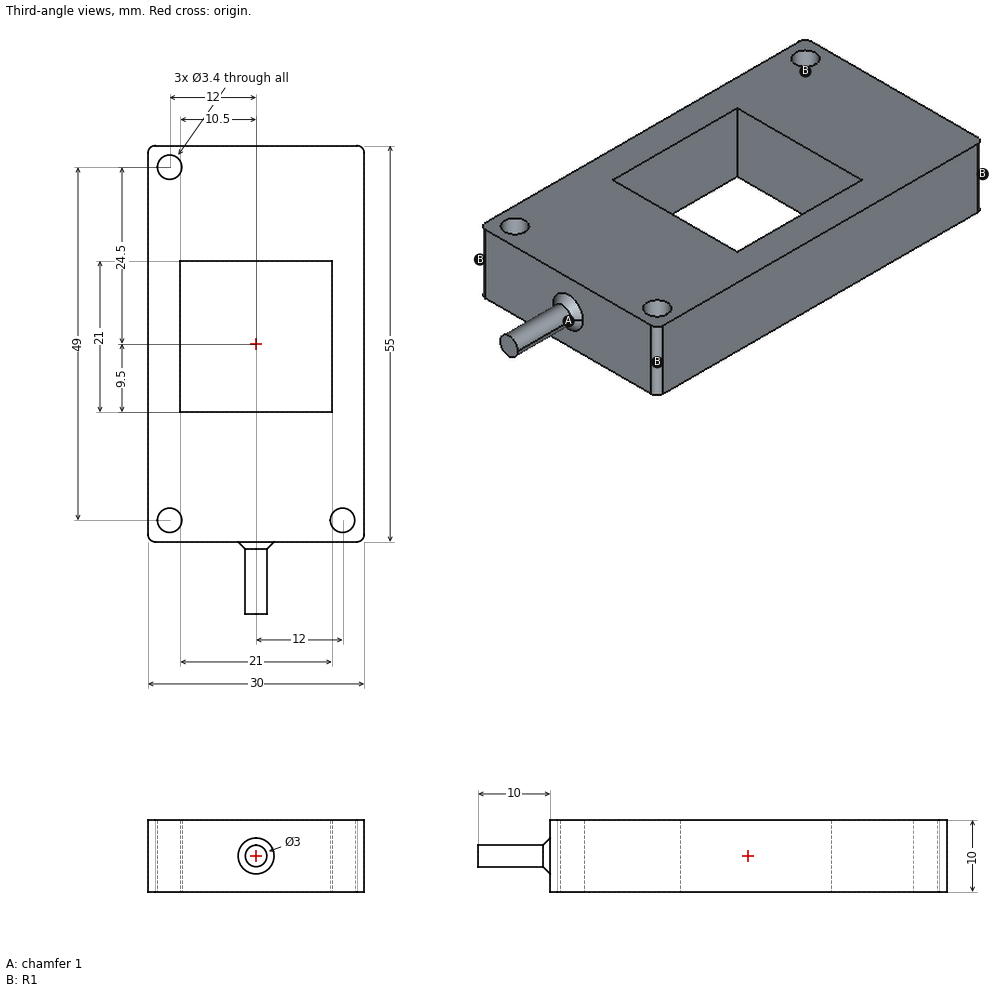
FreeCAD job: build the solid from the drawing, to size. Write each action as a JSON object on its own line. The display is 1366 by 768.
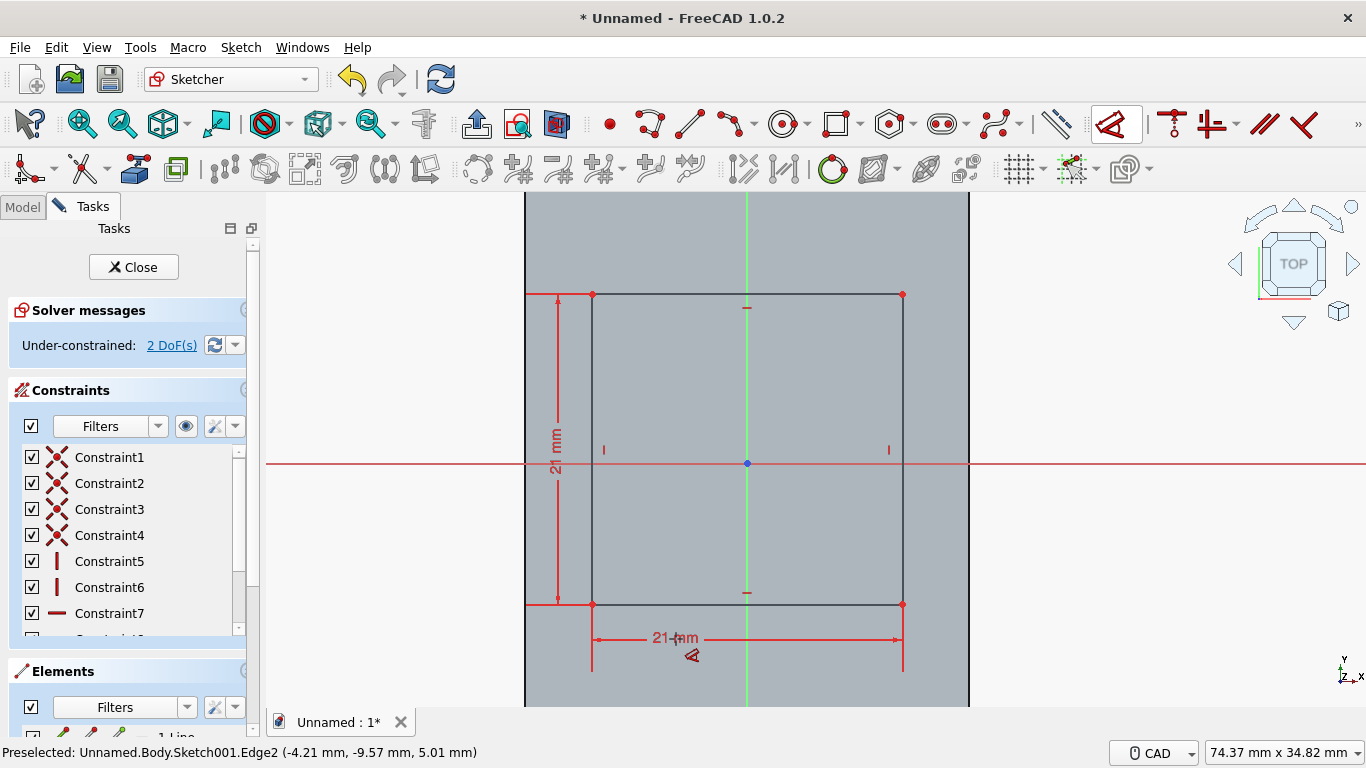
{"action": "left_click", "coordinate": [592, 605]}
{"action": "left_click", "coordinate": [558, 534]}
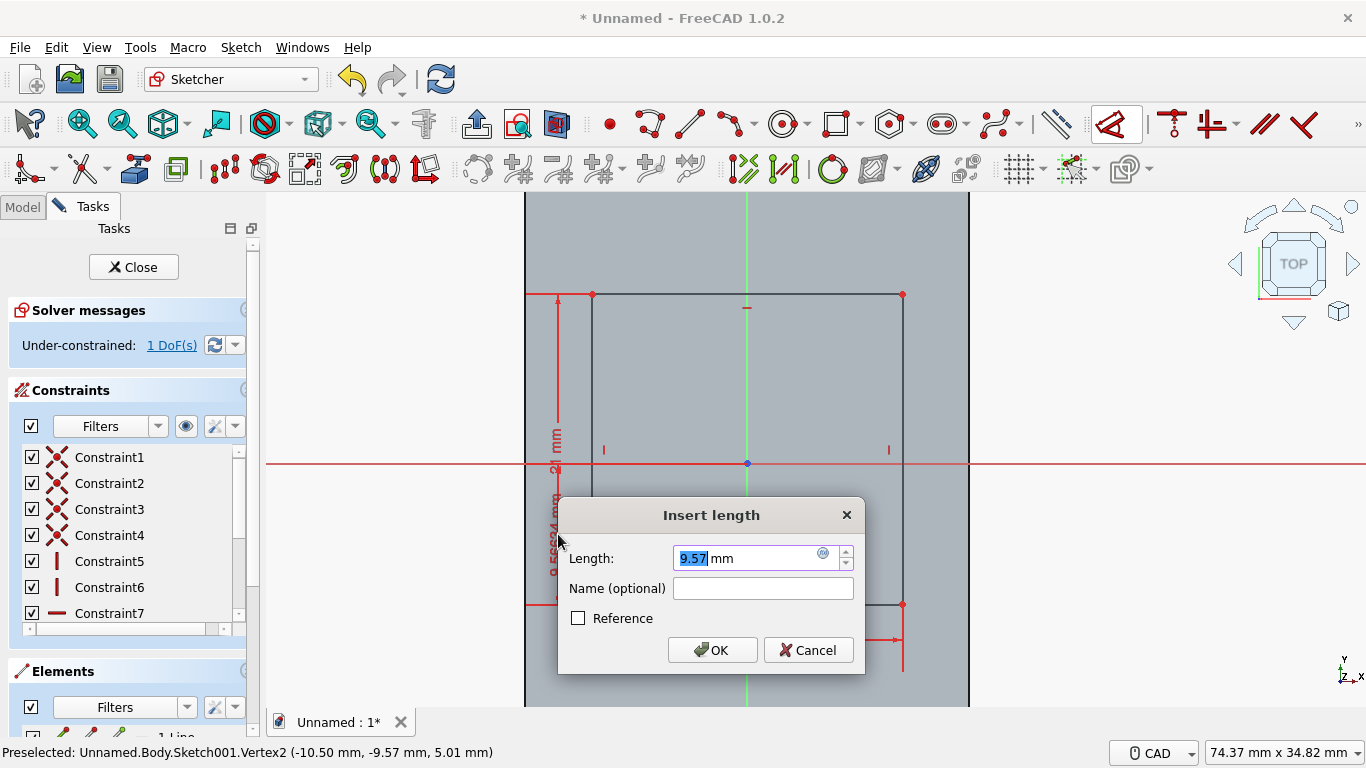
{"action": "type", "text": "9.5"}
{"action": "key", "text": "Return"}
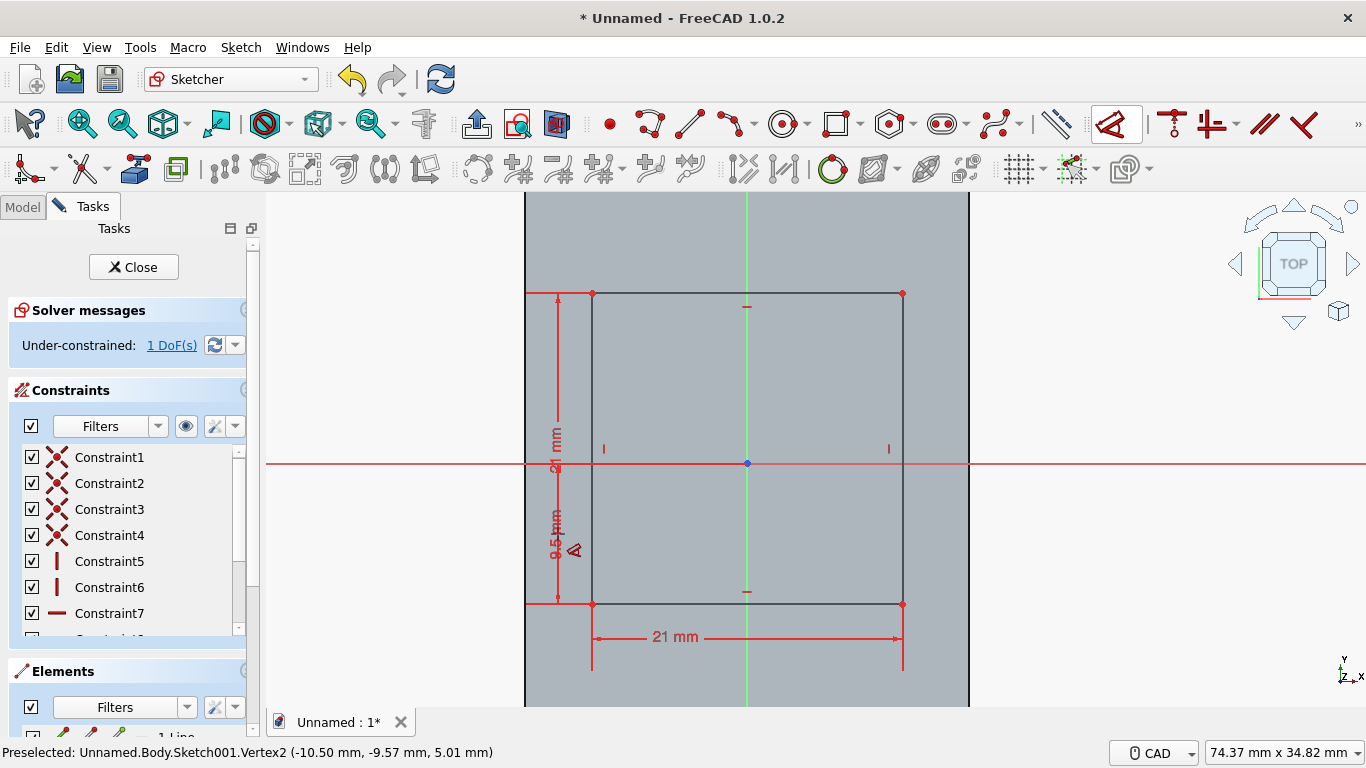
{"action": "left_click", "coordinate": [592, 293]}
{"action": "left_click", "coordinate": [670, 259]}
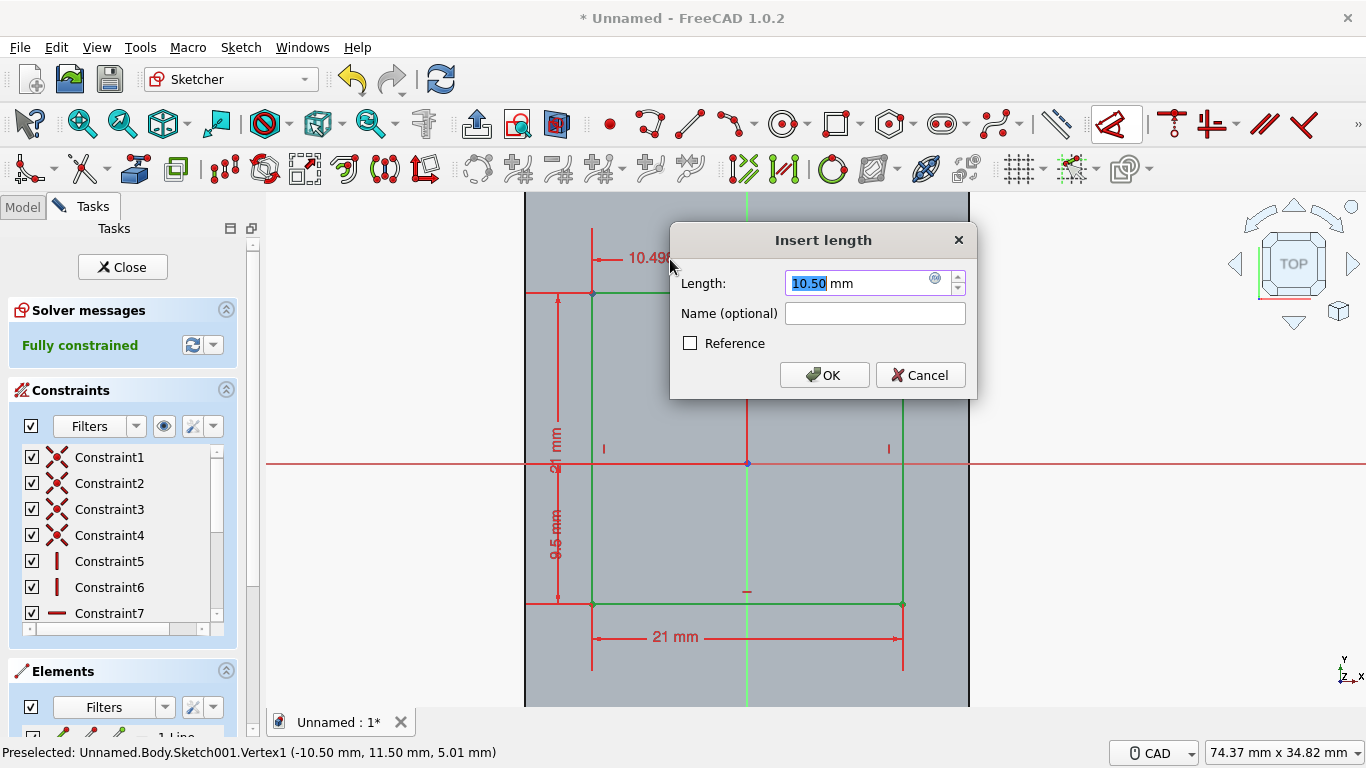
{"action": "type", "text": "10.5"}
{"action": "key", "text": "Return"}
{"action": "key", "text": "Escape"}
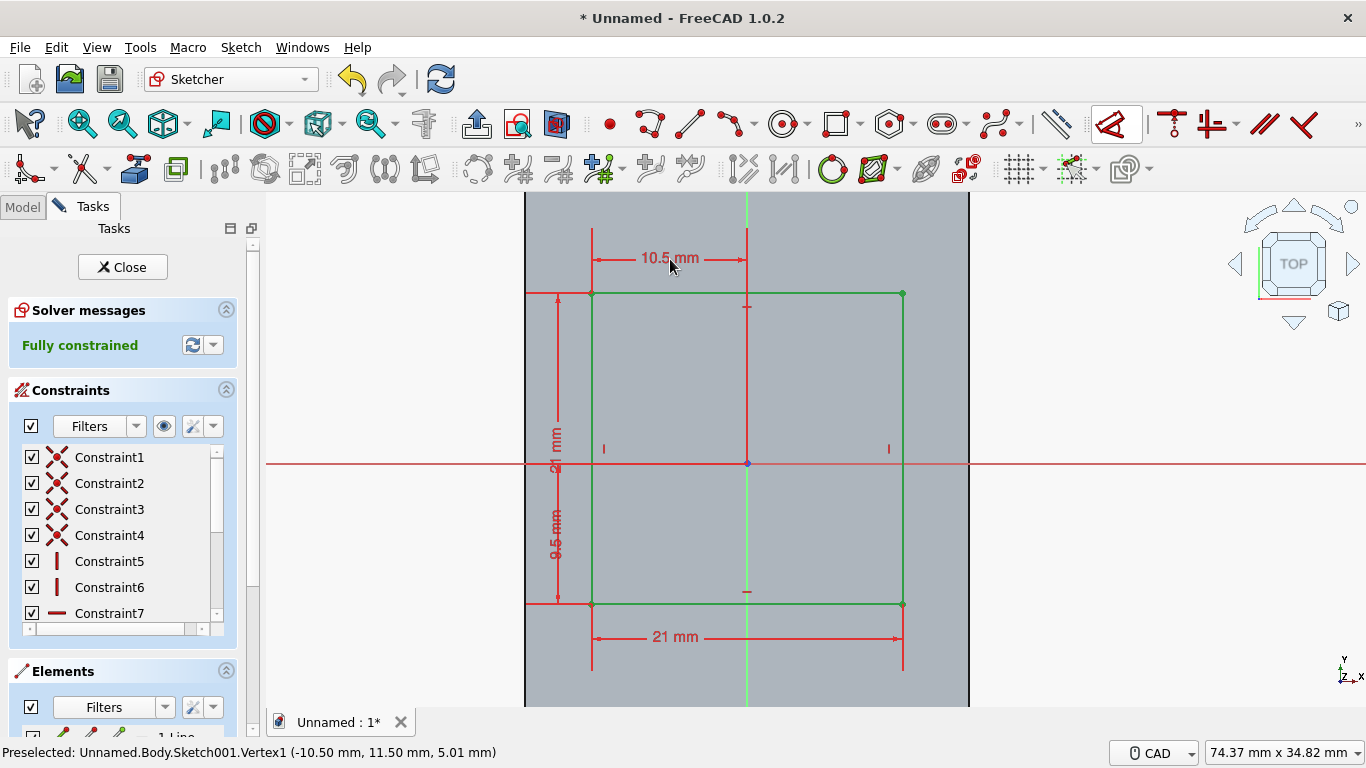
{"action": "left_click", "coordinate": [123, 267]}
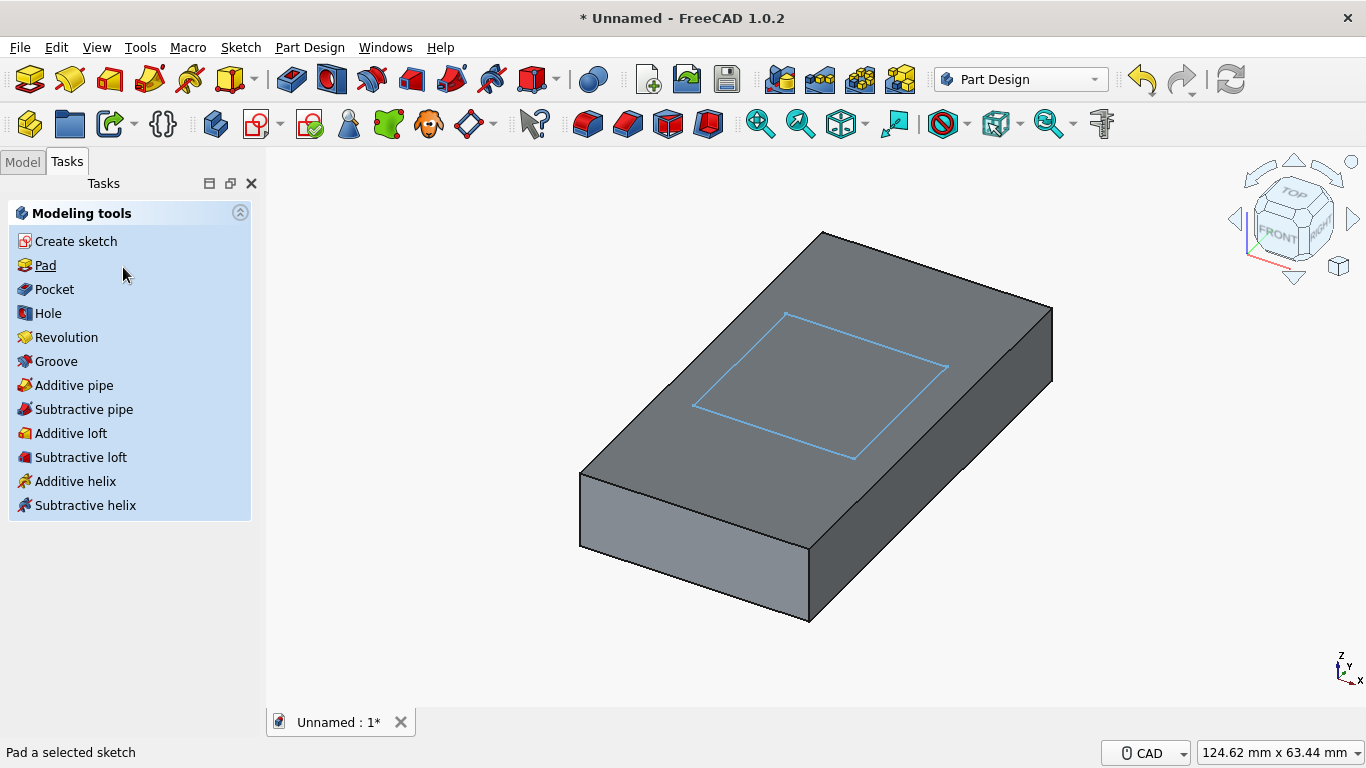
{"action": "left_click", "coordinate": [292, 80]}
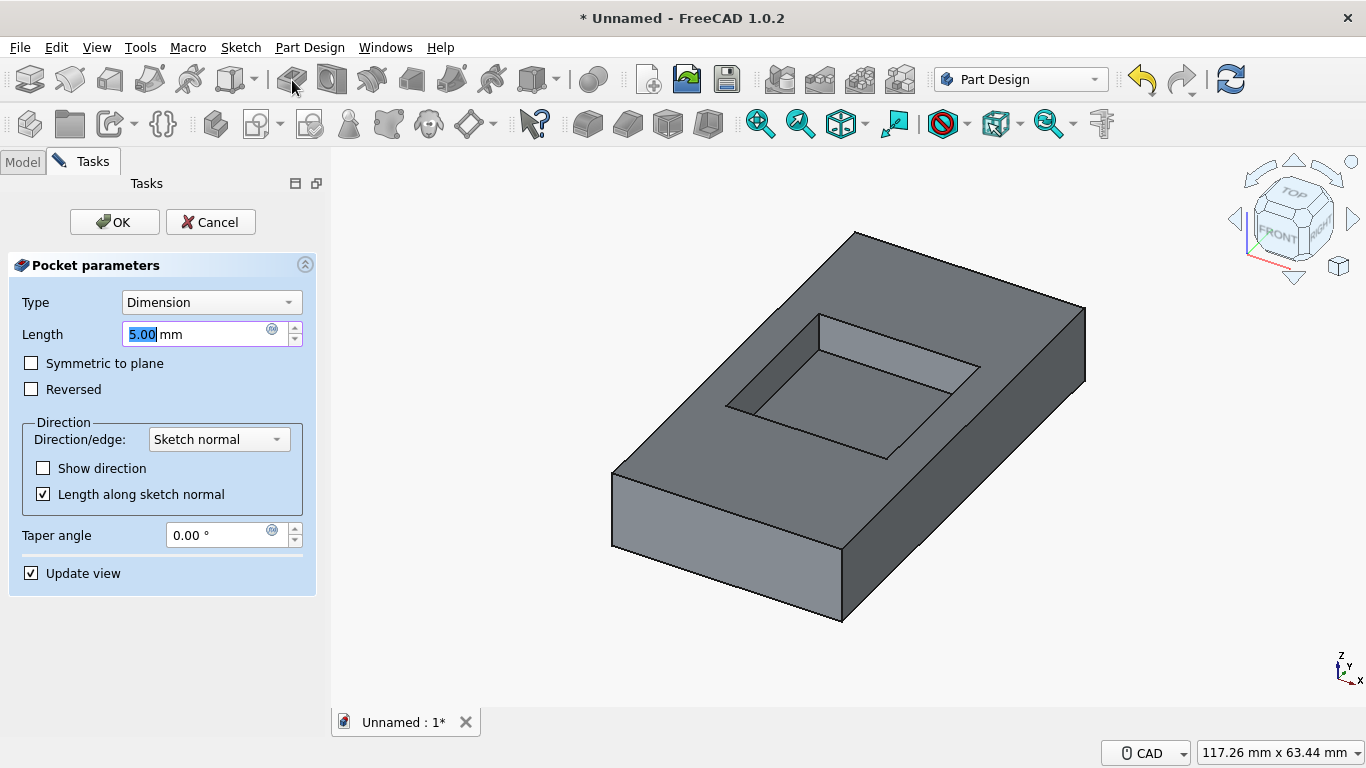
{"action": "left_click", "coordinate": [212, 302]}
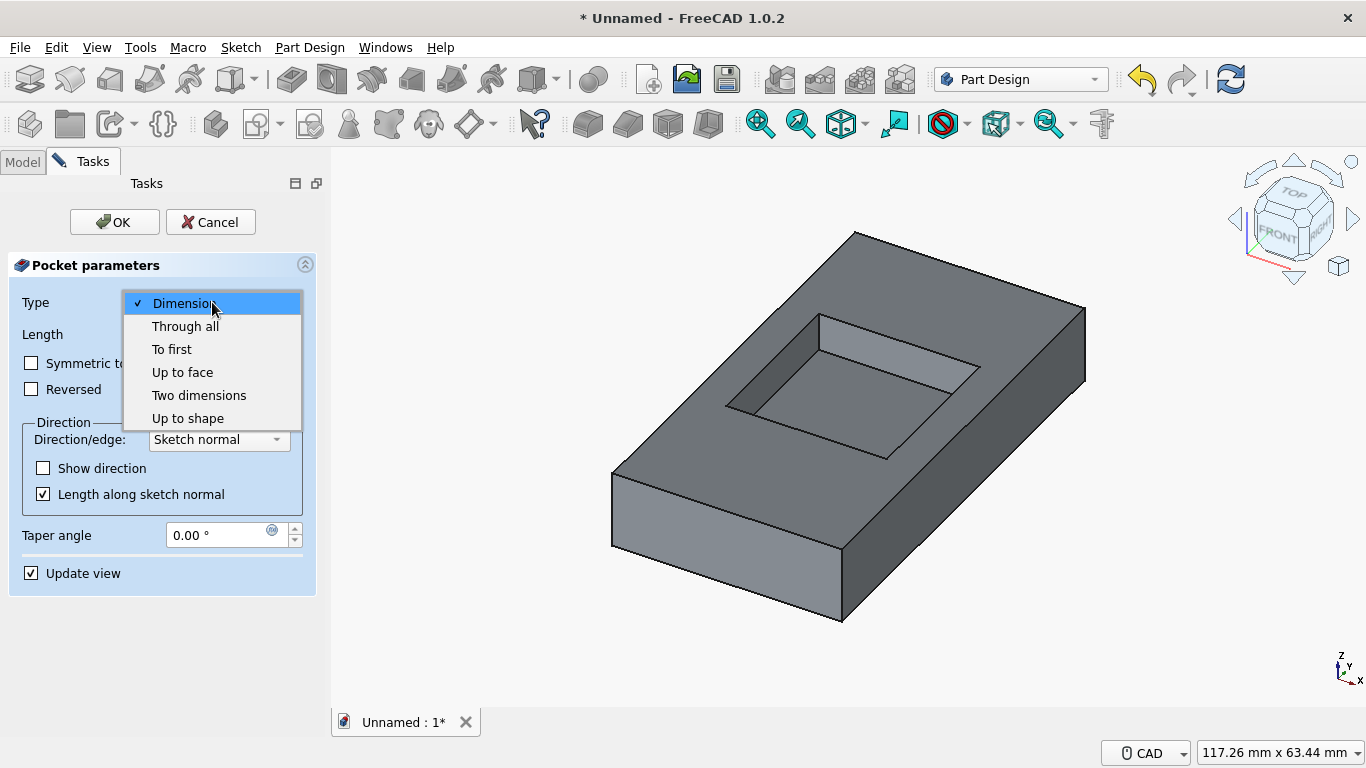
{"action": "left_click", "coordinate": [212, 326]}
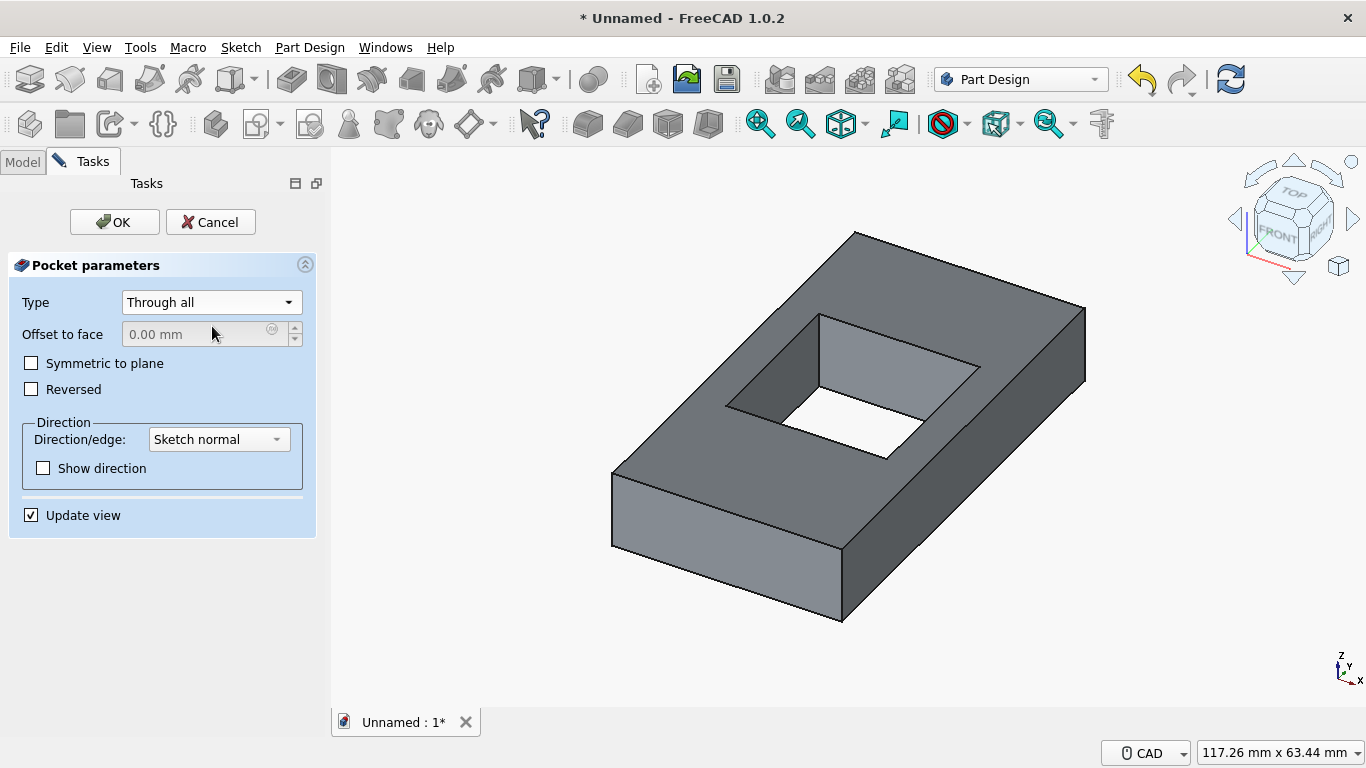
{"action": "left_click", "coordinate": [115, 222]}